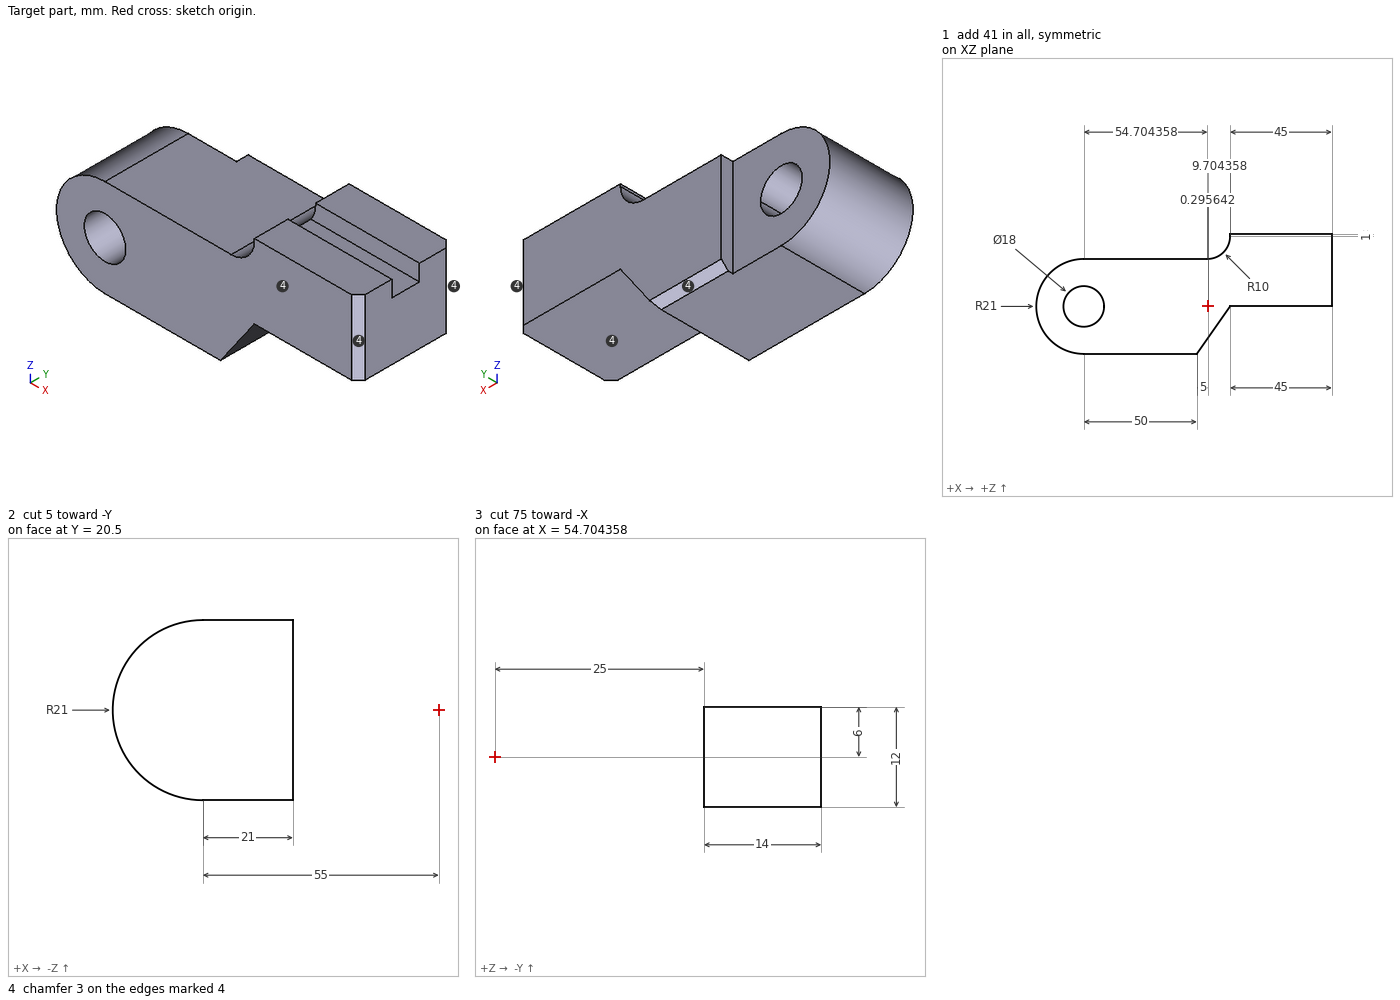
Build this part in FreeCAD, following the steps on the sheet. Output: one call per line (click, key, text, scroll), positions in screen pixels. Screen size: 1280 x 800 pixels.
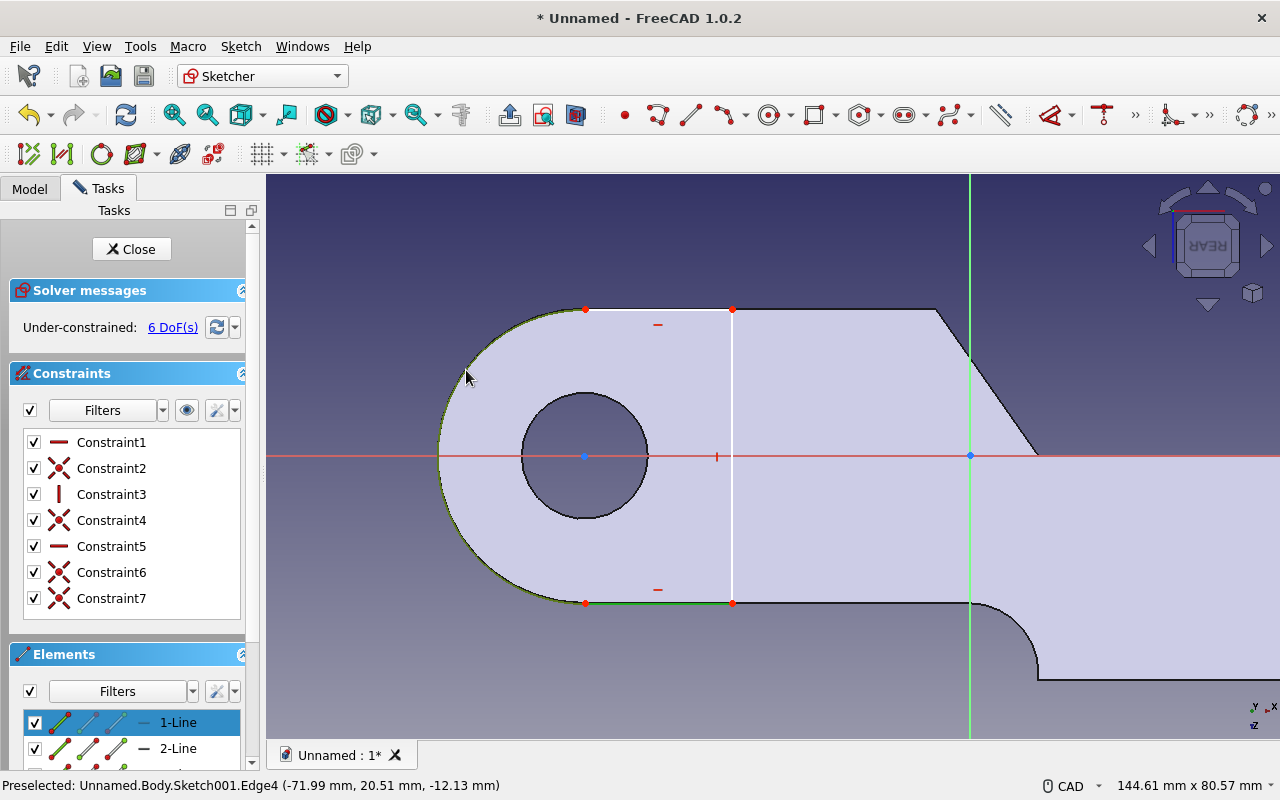
key(t)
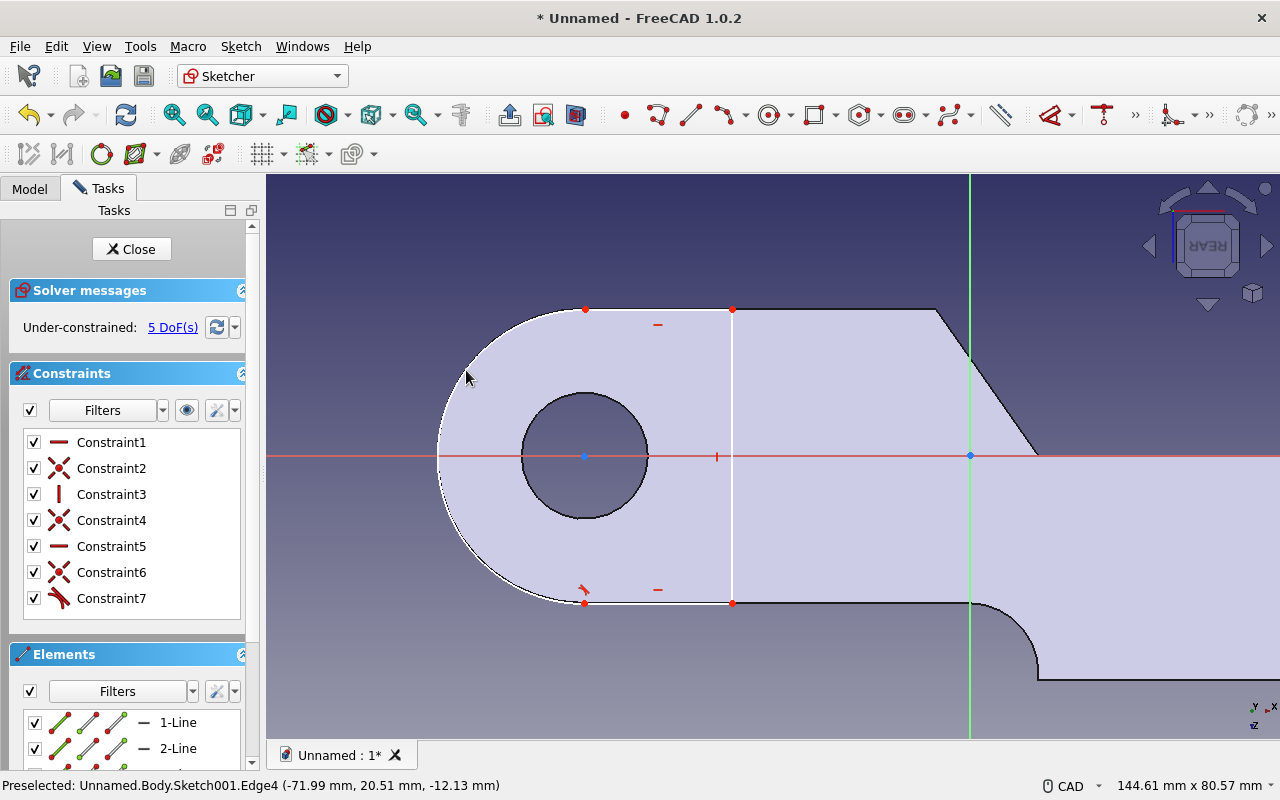
click(688, 310)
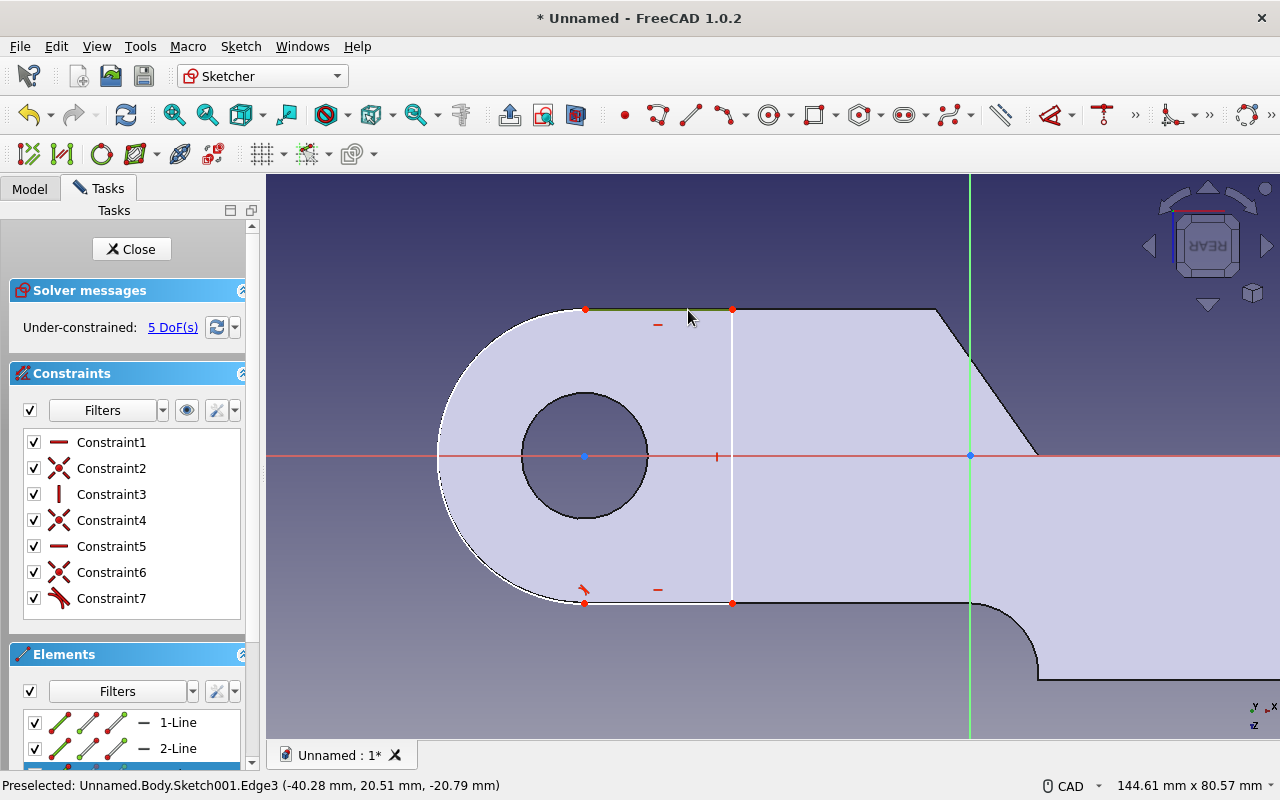
click(466, 370)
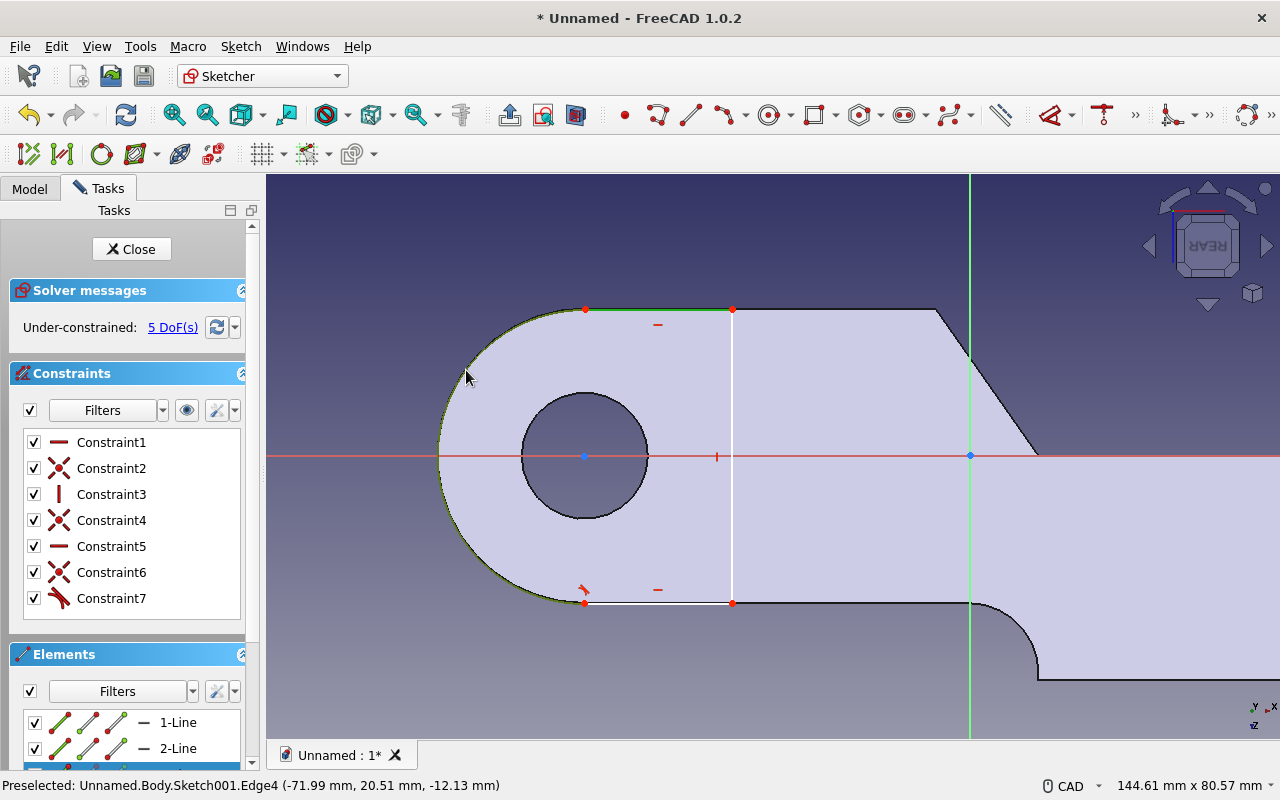
key(t)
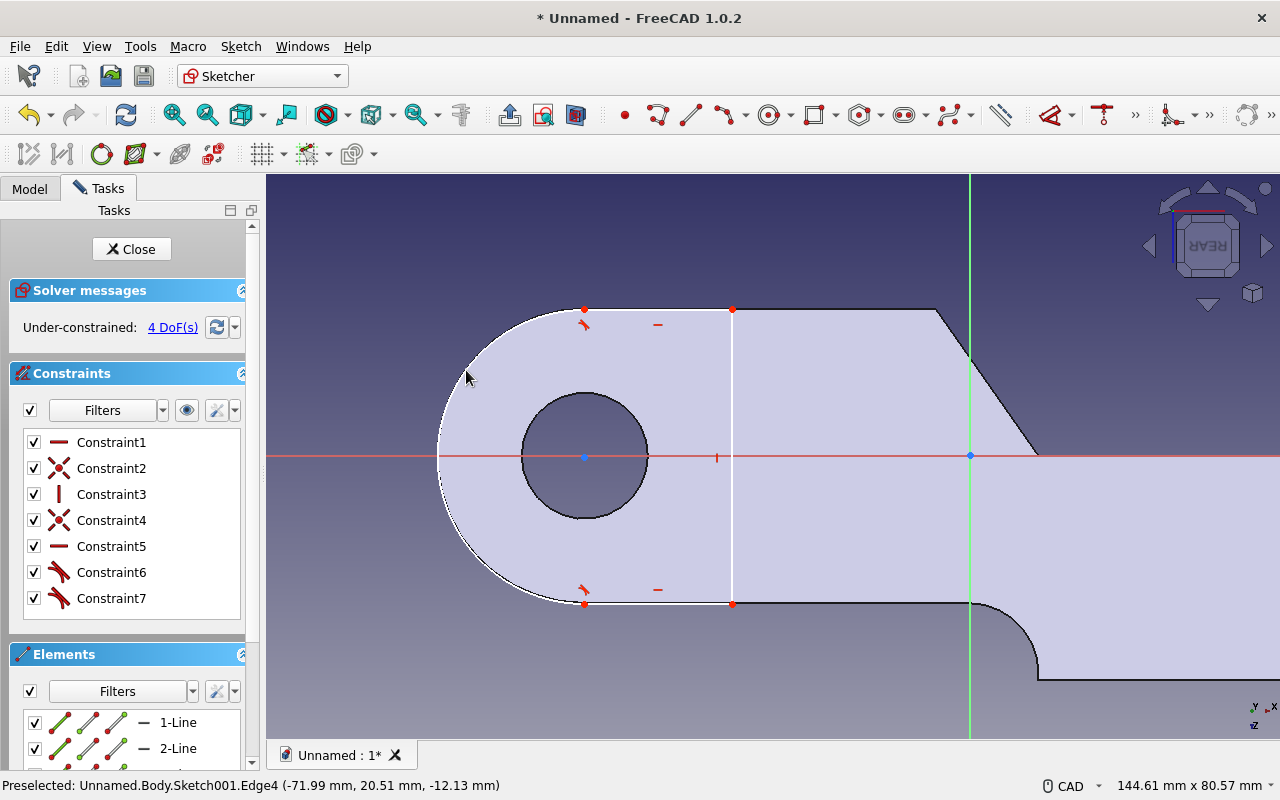
click(585, 457)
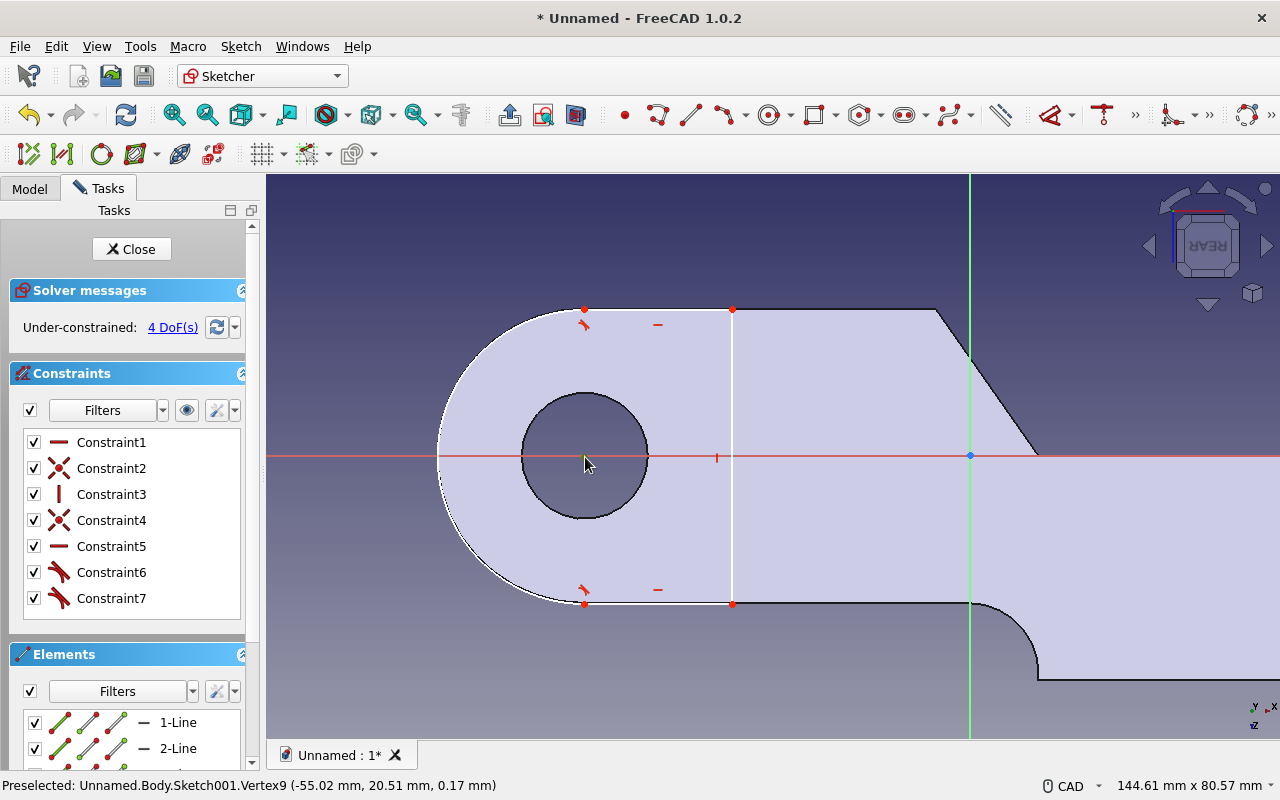
click(353, 456)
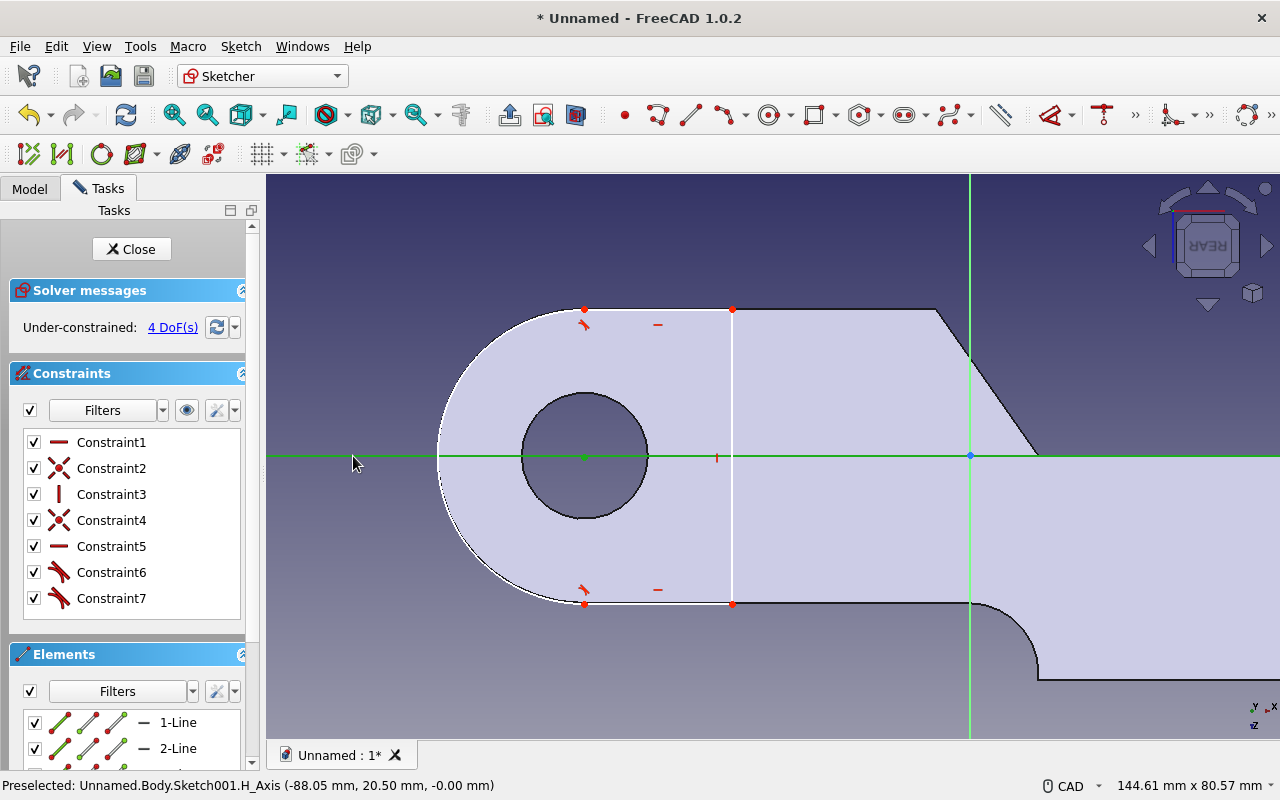
click(1102, 116)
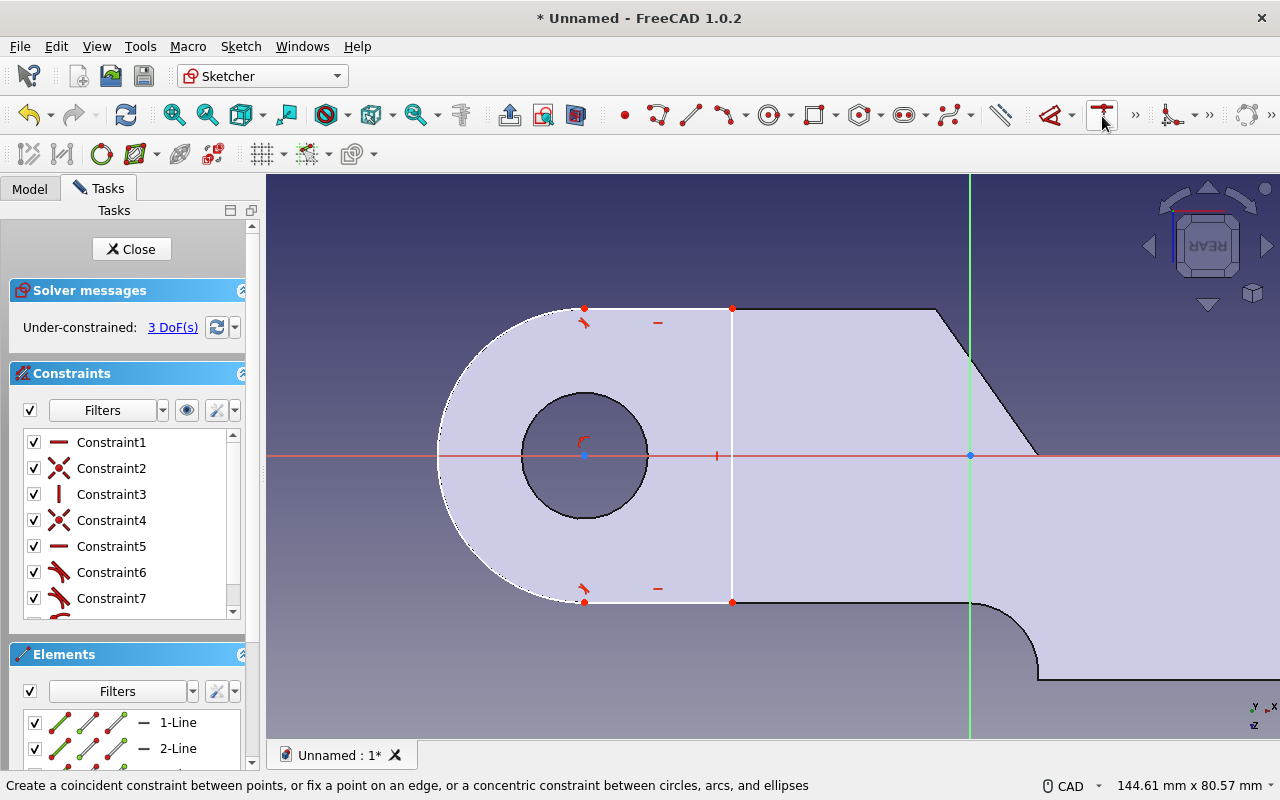
click(1050, 116)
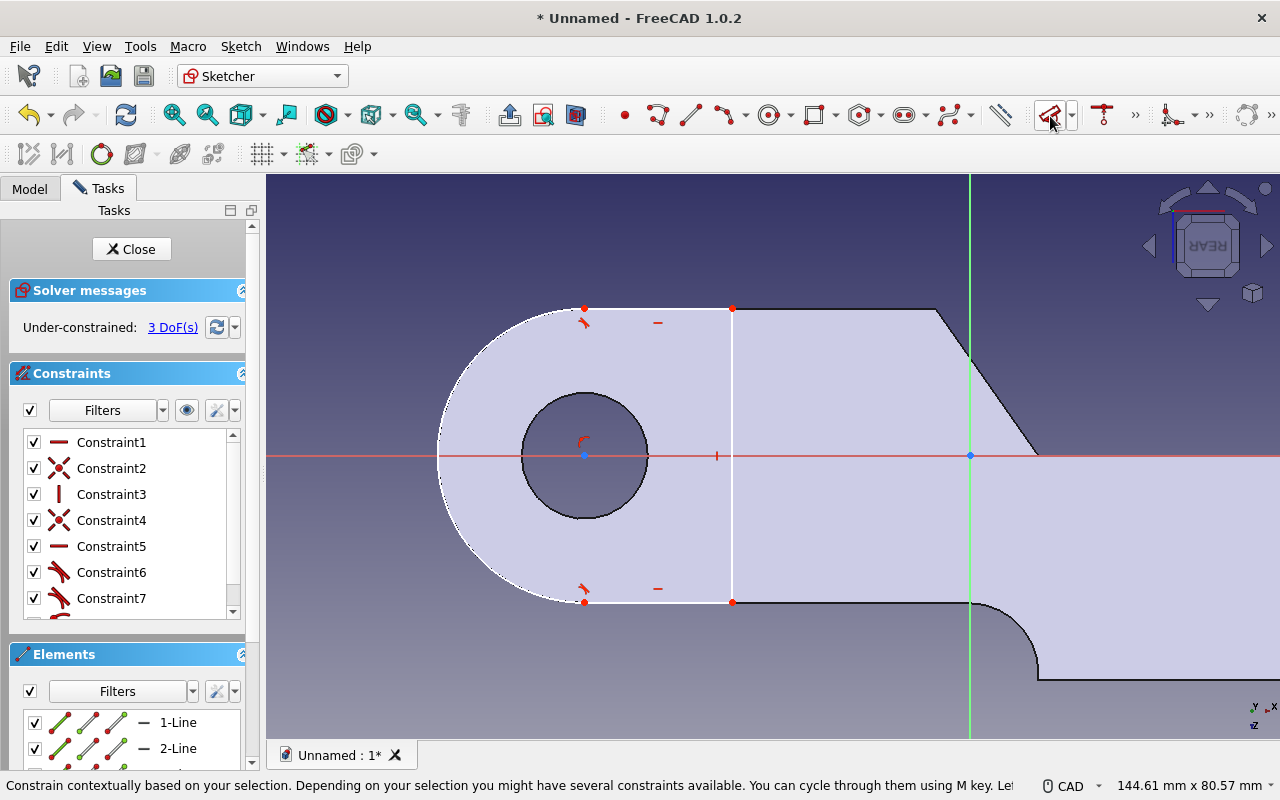
click(466, 369)
click(440, 350)